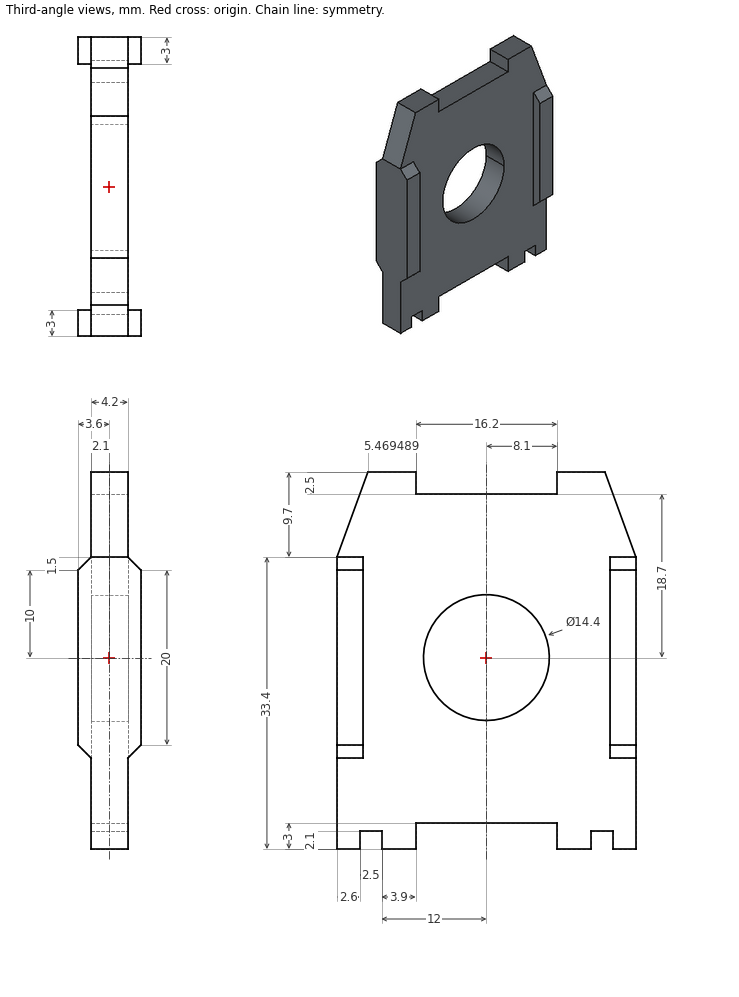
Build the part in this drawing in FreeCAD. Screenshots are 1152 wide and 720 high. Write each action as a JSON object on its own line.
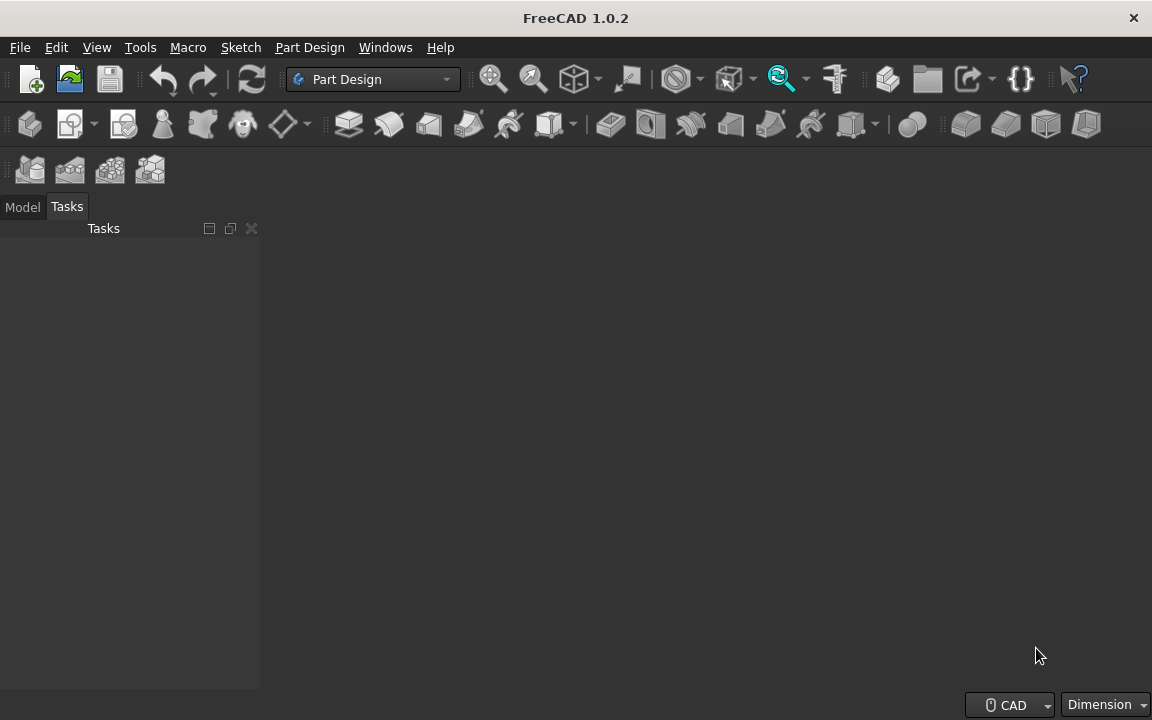
{"action": "left_click", "coordinate": [30, 80]}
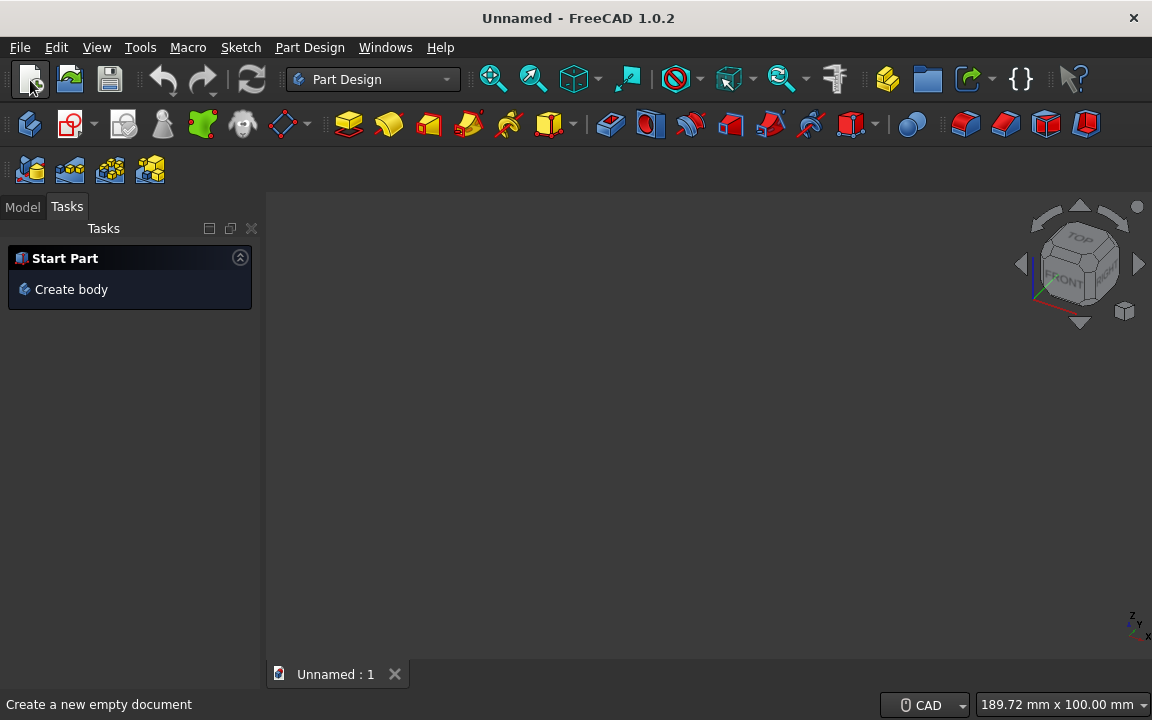
{"action": "left_click", "coordinate": [70, 124]}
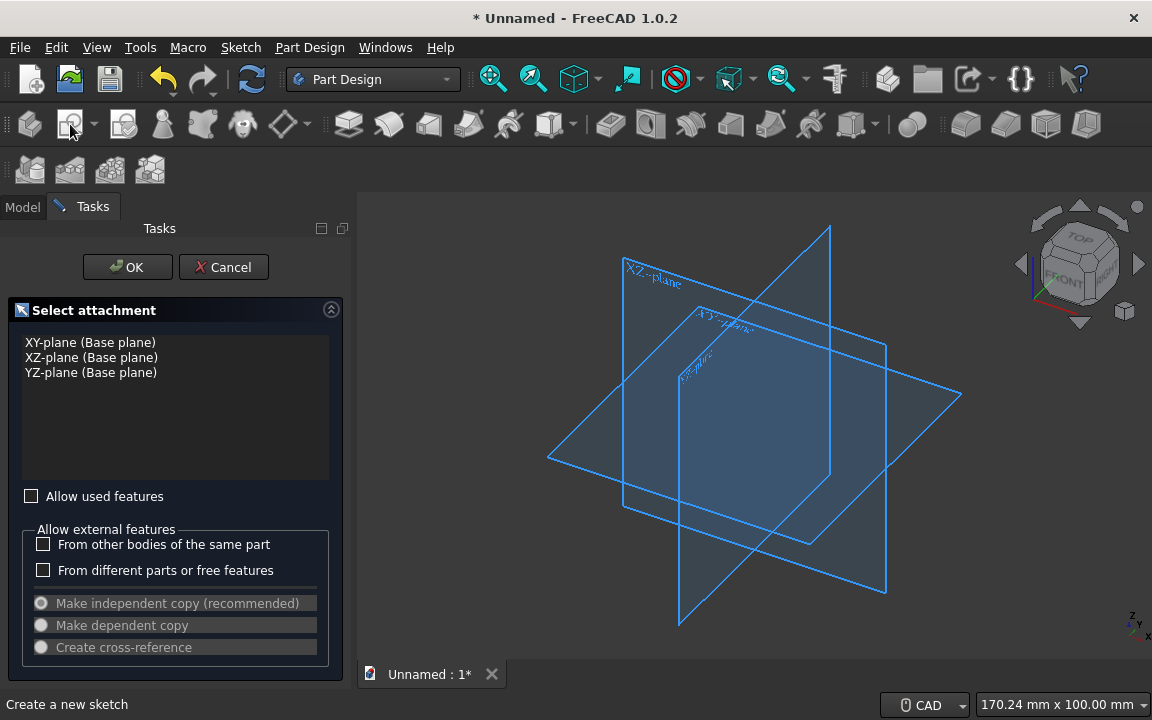
{"action": "left_click", "coordinate": [82, 372]}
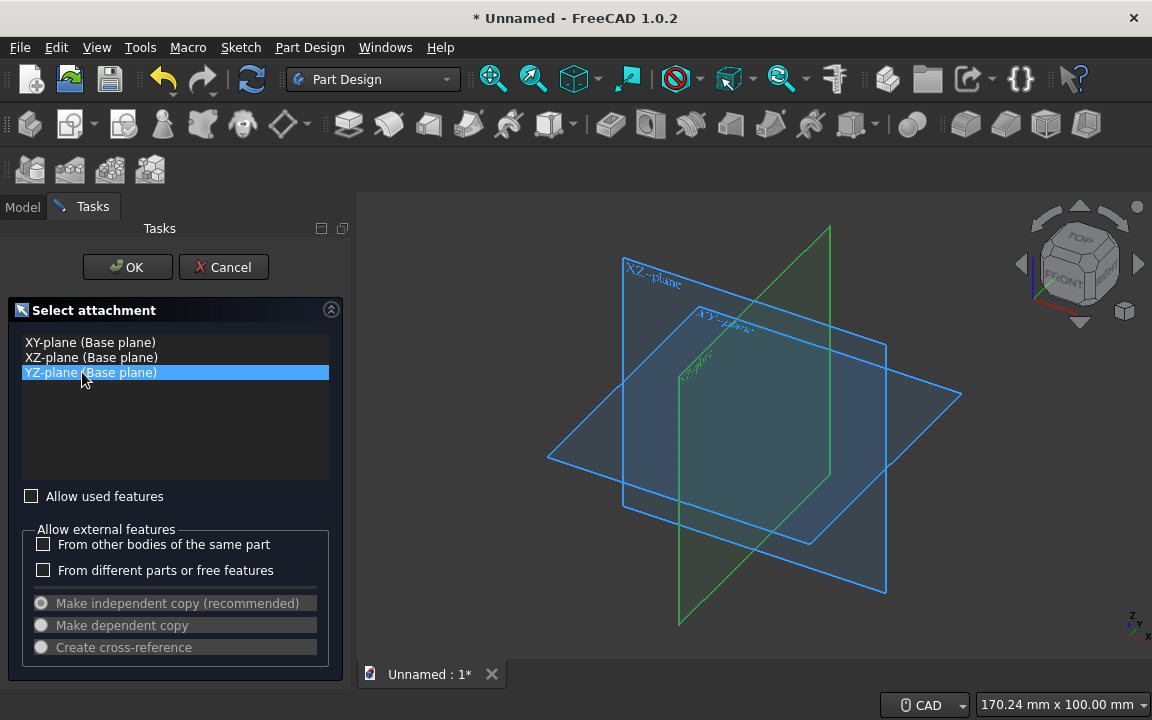
{"action": "left_click", "coordinate": [128, 267]}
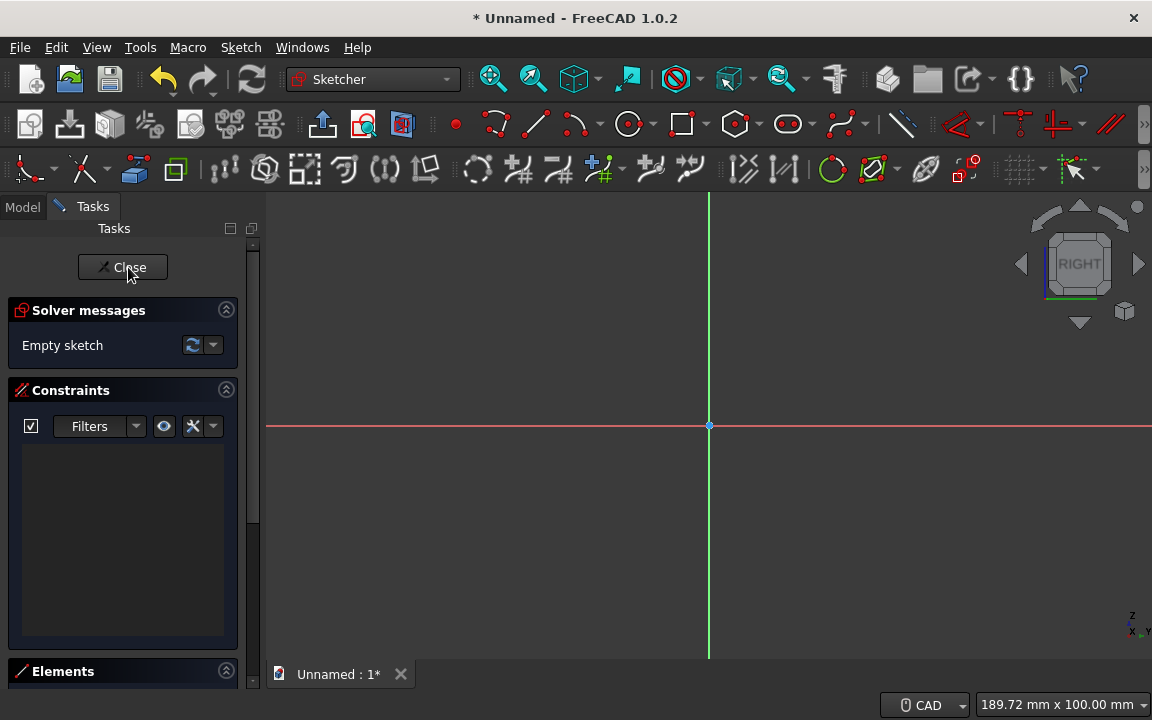
{"action": "scroll", "coordinate": [848, 430], "scroll_direction": "up", "scroll_amount": 2}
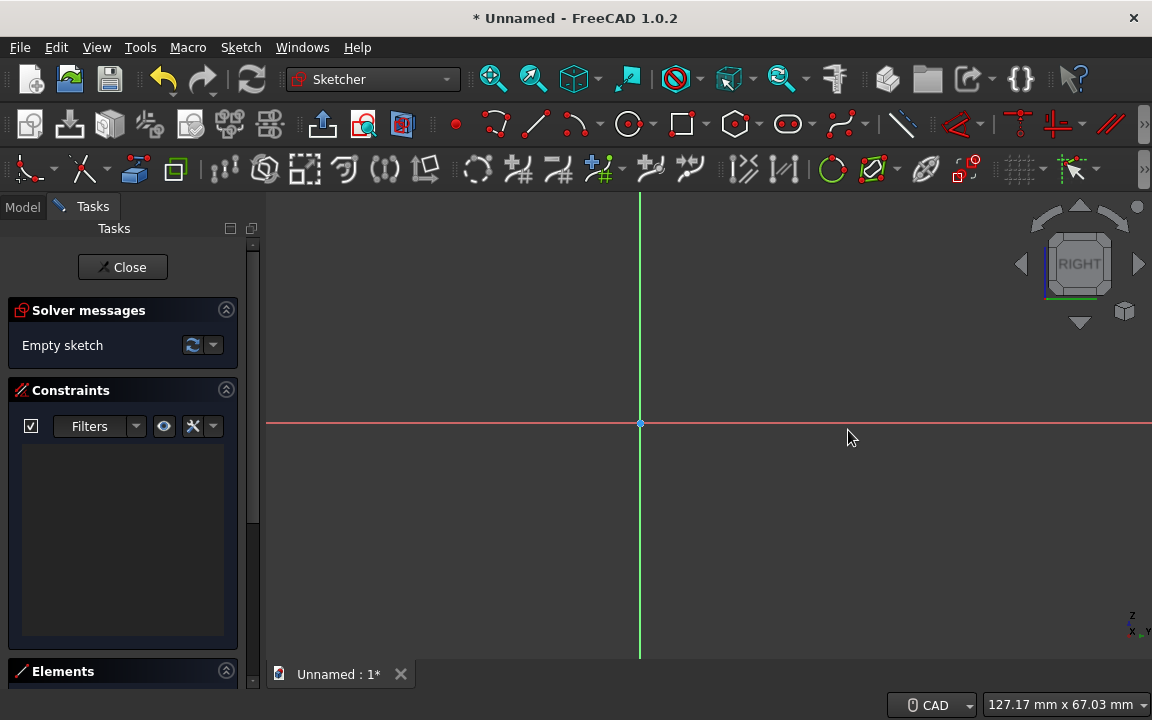
{"action": "left_click", "coordinate": [496, 124]}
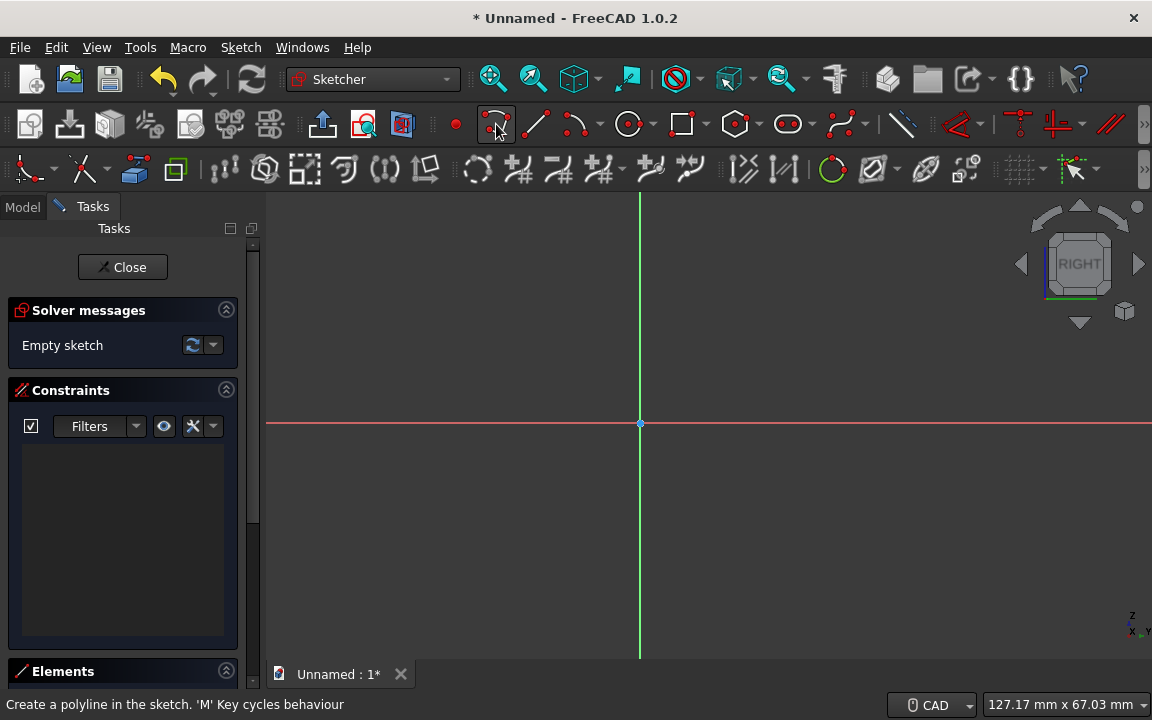
{"action": "left_click", "coordinate": [697, 293]}
{"action": "left_click", "coordinate": [584, 293]}
{"action": "left_click", "coordinate": [584, 275]}
{"action": "left_click", "coordinate": [546, 275]}
{"action": "left_click", "coordinate": [521, 343]}
{"action": "left_click", "coordinate": [521, 576]}
{"action": "left_click", "coordinate": [539, 576]}
{"action": "left_click", "coordinate": [539, 561]}
{"action": "left_click", "coordinate": [557, 561]}
{"action": "left_click", "coordinate": [557, 576]}
{"action": "left_click", "coordinate": [584, 576]}
{"action": "left_click", "coordinate": [584, 555]}
{"action": "left_click", "coordinate": [697, 555]}
{"action": "left_click", "coordinate": [697, 576]}
{"action": "left_click", "coordinate": [724, 576]}
{"action": "left_click", "coordinate": [724, 561]}
{"action": "left_click", "coordinate": [741, 561]}
{"action": "left_click", "coordinate": [741, 576]}
{"action": "left_click", "coordinate": [759, 576]}
{"action": "left_click", "coordinate": [759, 343]}
{"action": "left_click", "coordinate": [735, 275]}
{"action": "left_click", "coordinate": [697, 275]}
{"action": "left_click", "coordinate": [697, 294]}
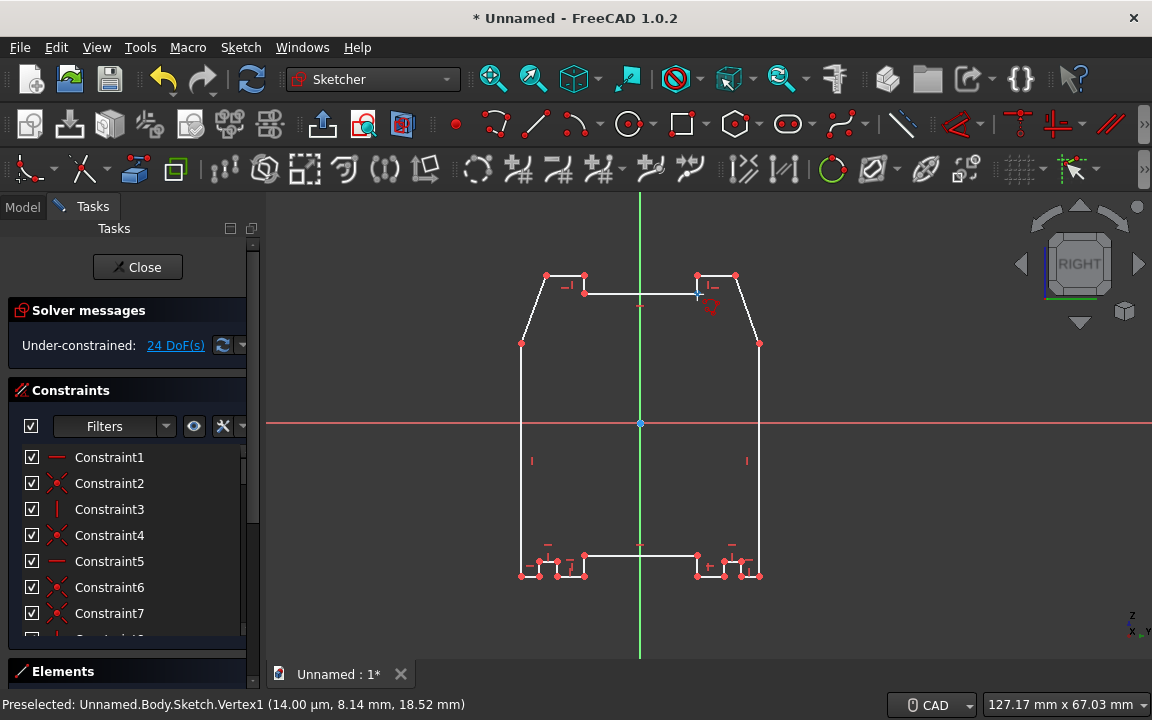
{"action": "left_click", "coordinate": [630, 124]}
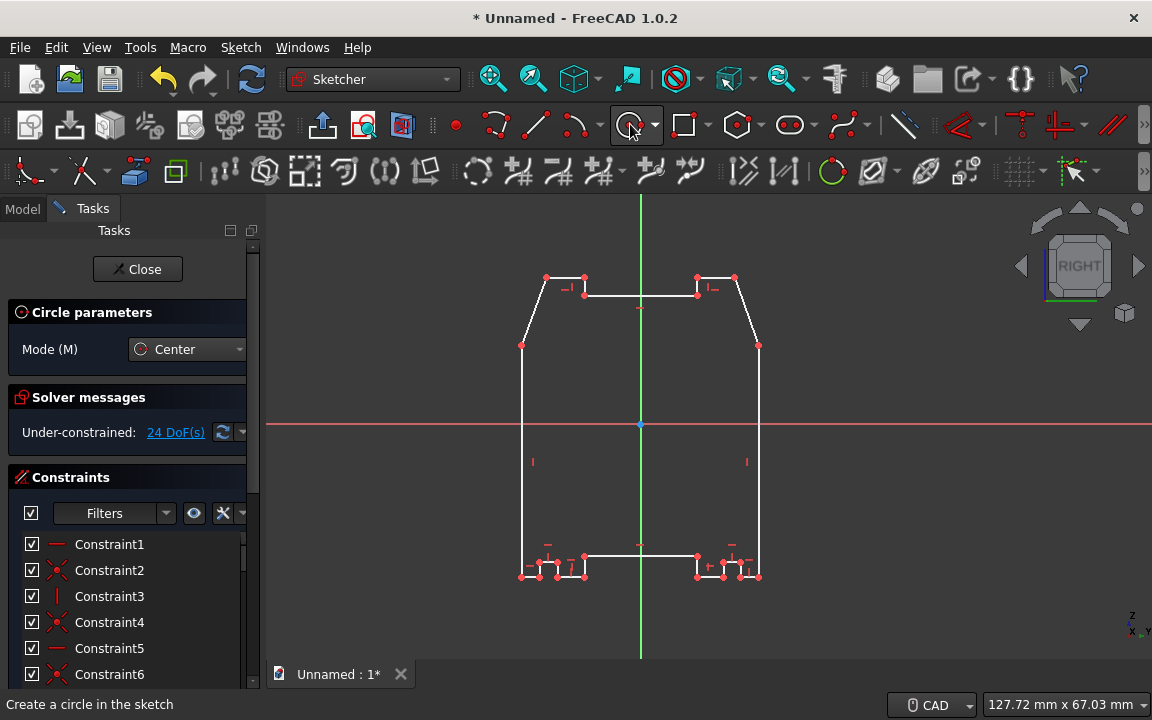
{"action": "left_click", "coordinate": [641, 424]}
{"action": "mouse_move", "coordinate": [676, 389]}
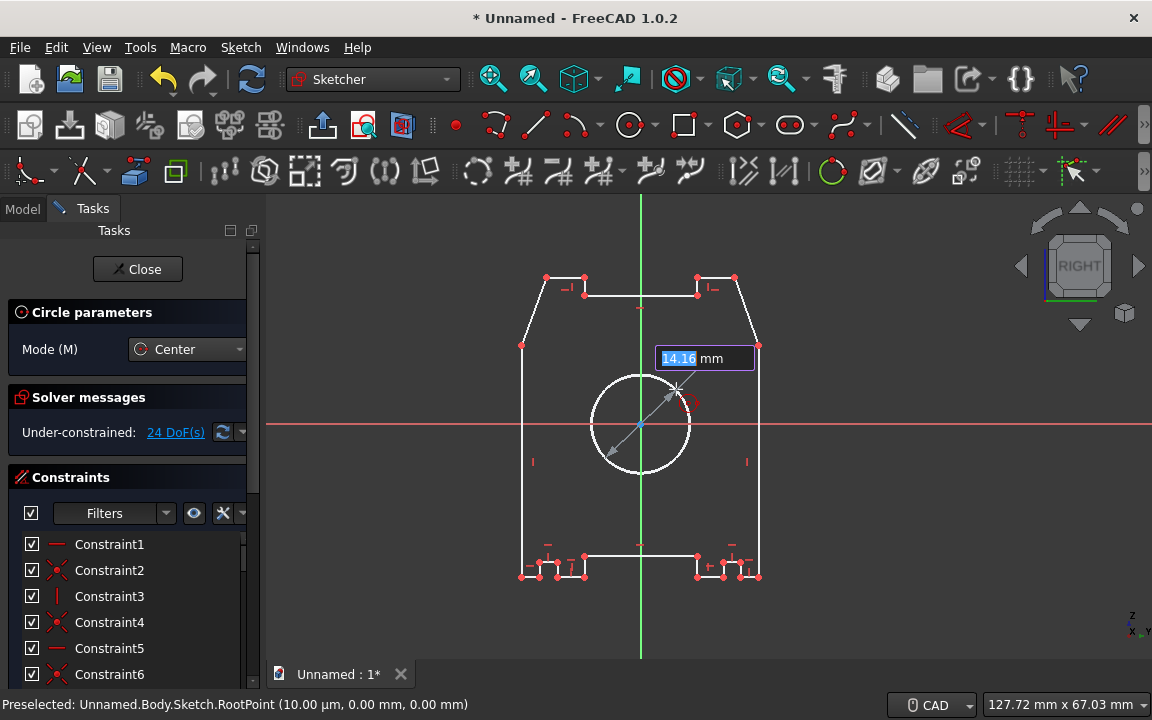
{"action": "type", "text": "14.4"}
{"action": "key", "text": "Return"}
{"action": "key", "text": "Escape"}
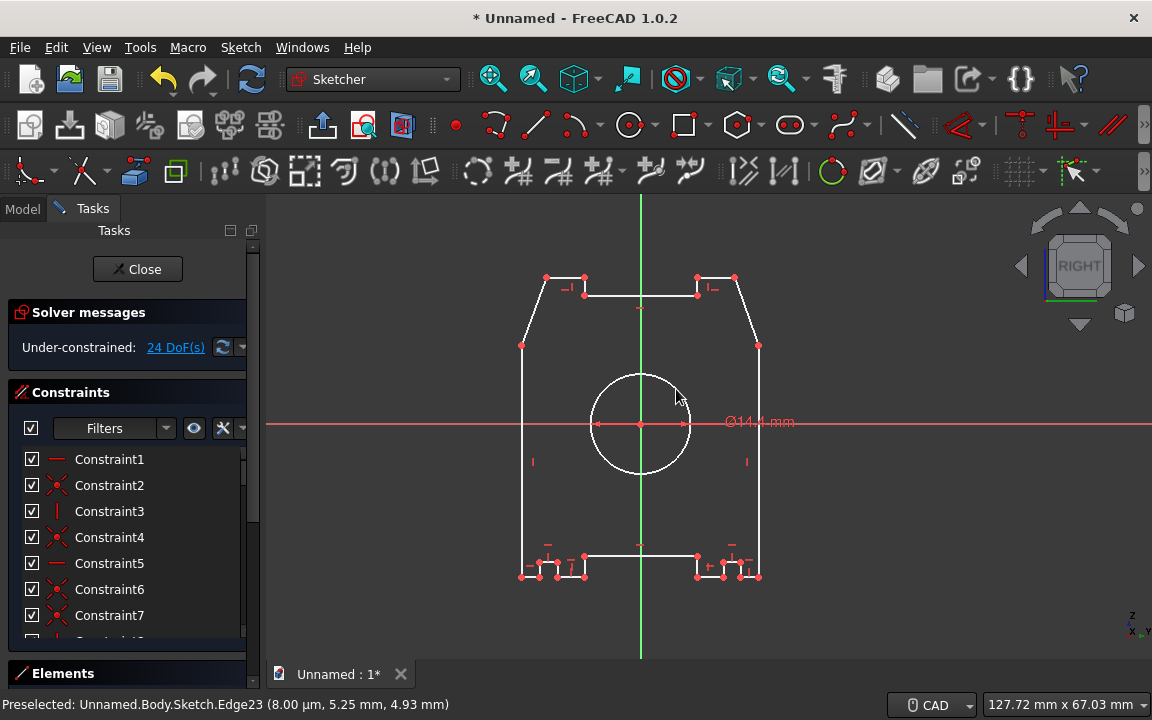
{"action": "left_click", "coordinate": [585, 577]}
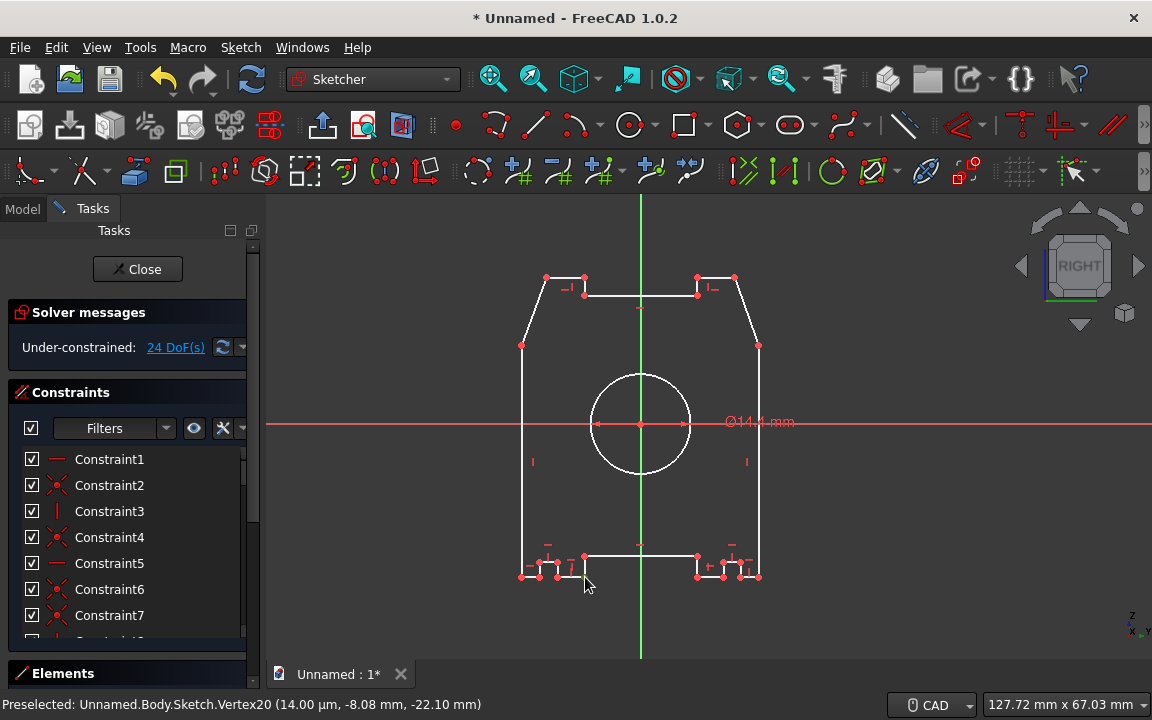
{"action": "left_click", "coordinate": [697, 577]}